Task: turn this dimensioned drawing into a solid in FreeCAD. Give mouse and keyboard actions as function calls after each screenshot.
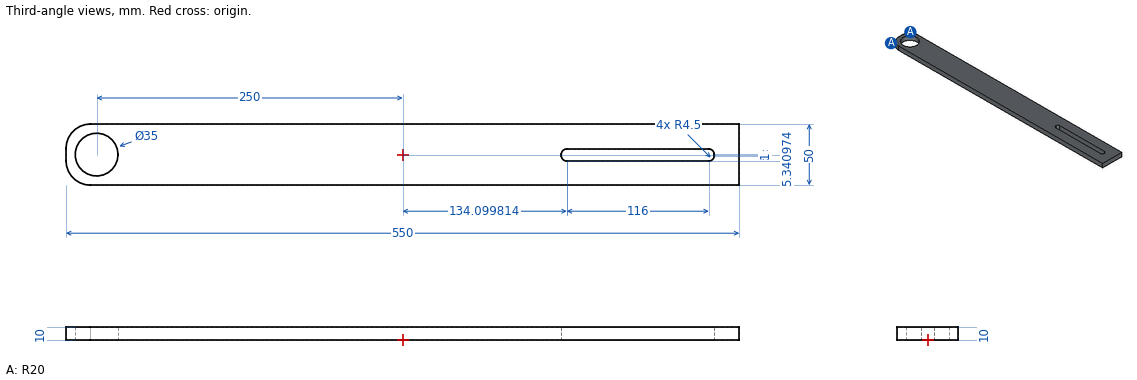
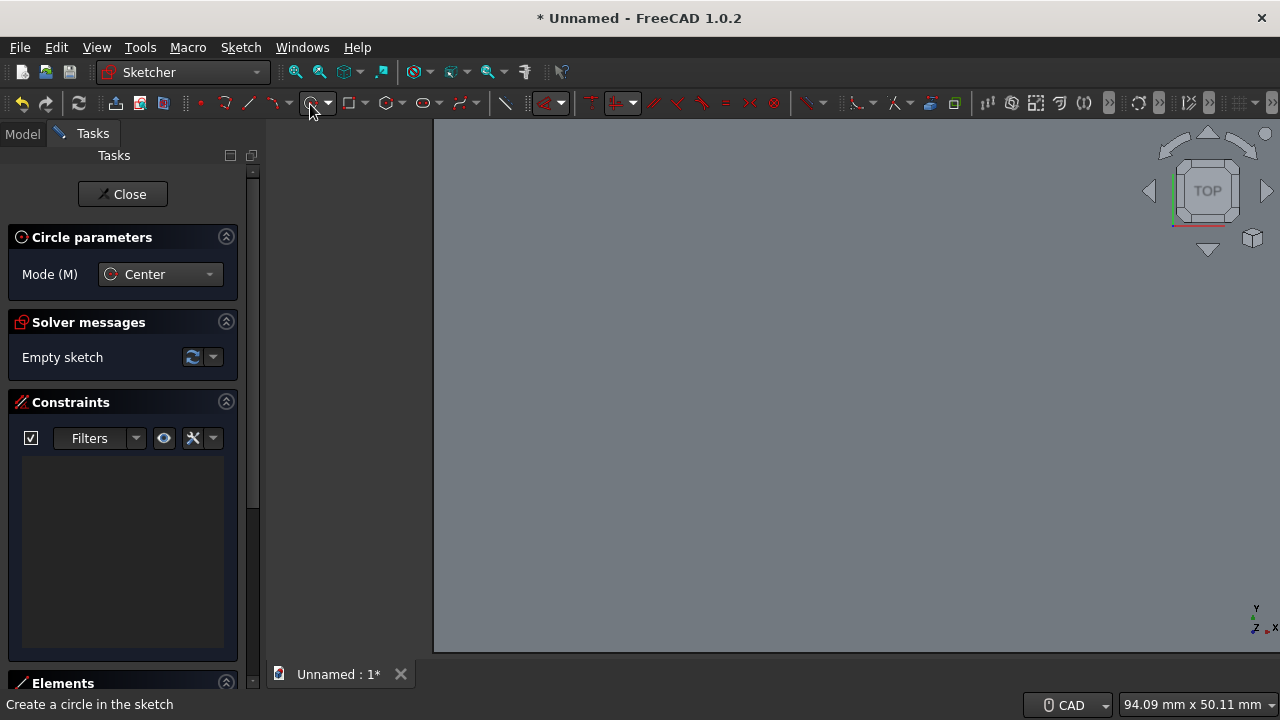
click(703, 384)
click(836, 251)
key(Escape)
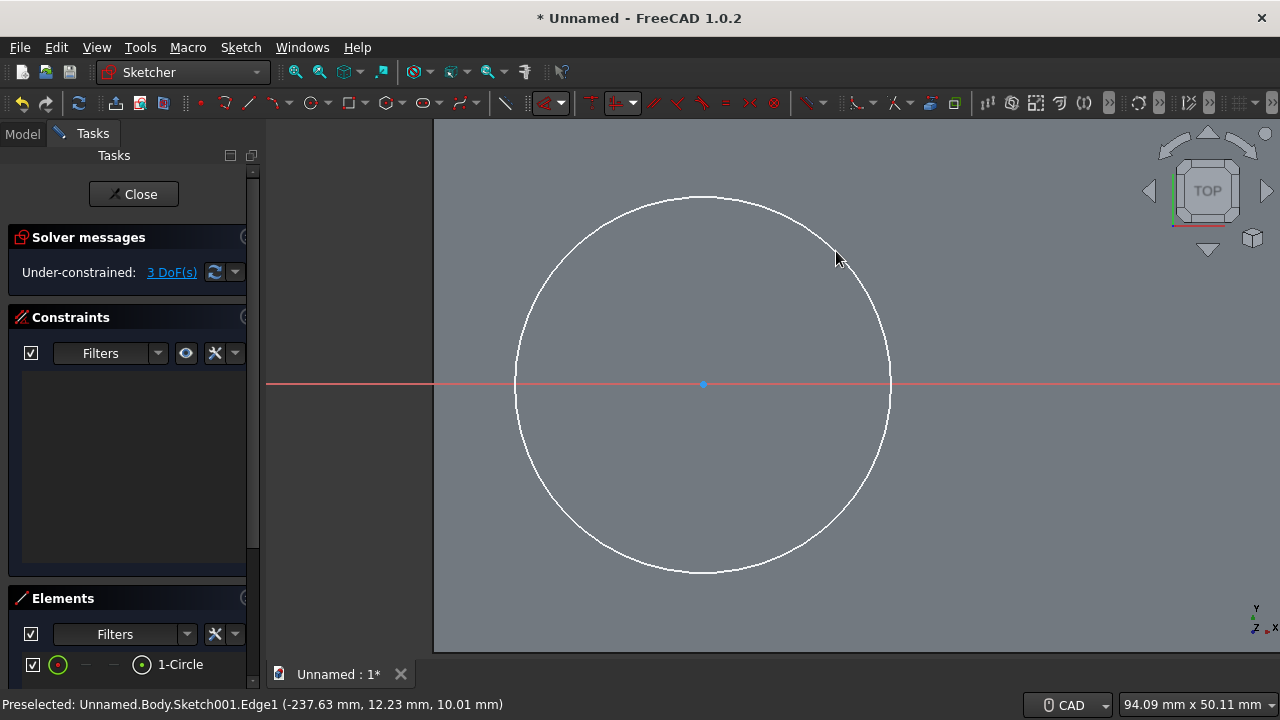
click(703, 385)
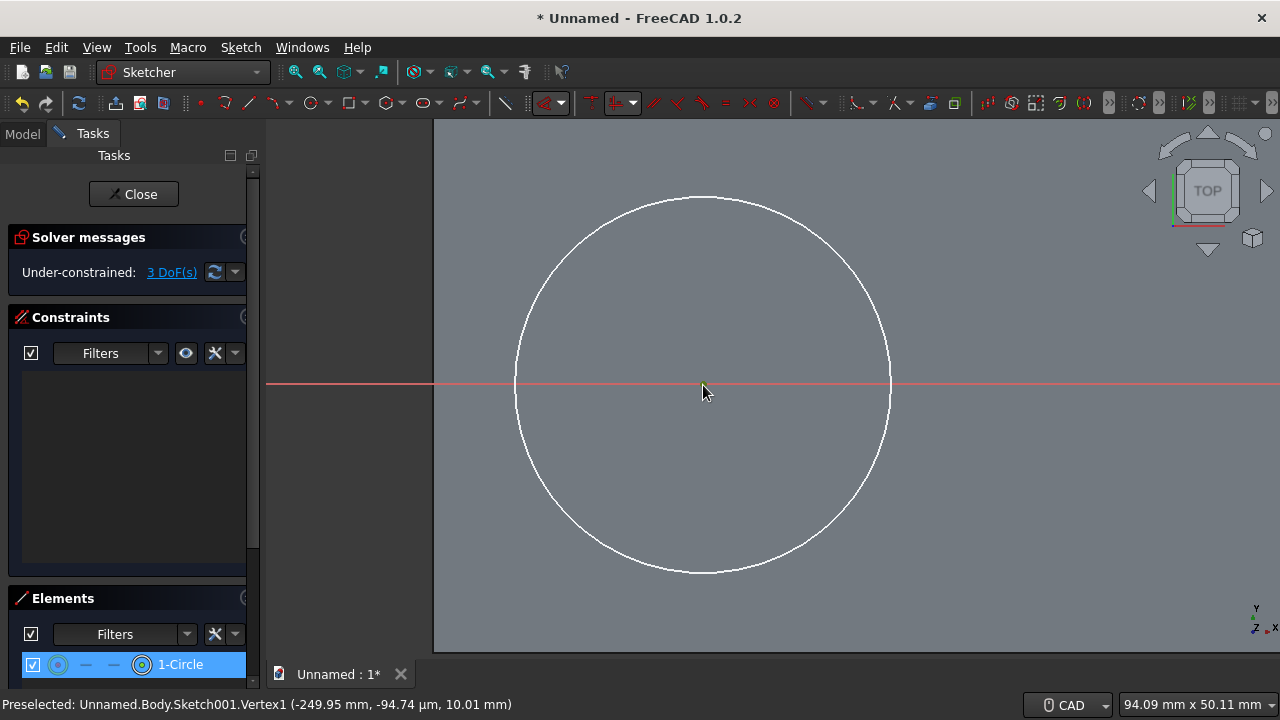
click(353, 384)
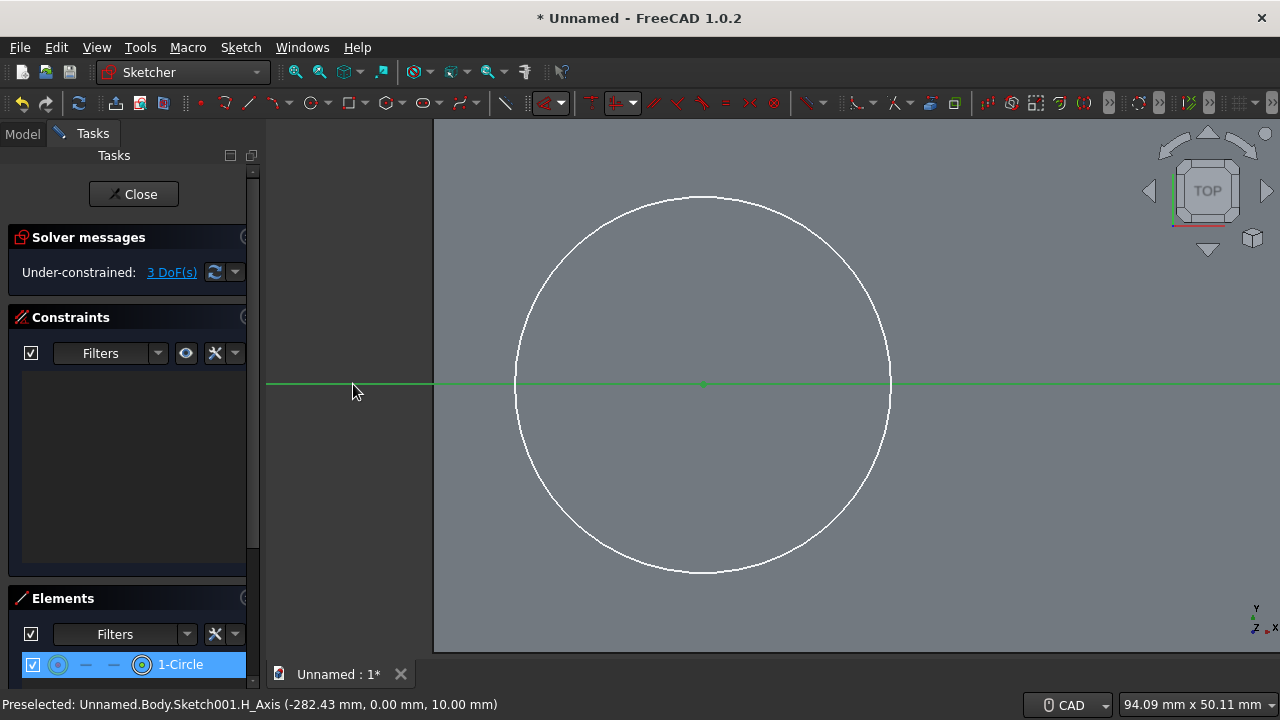
key(c)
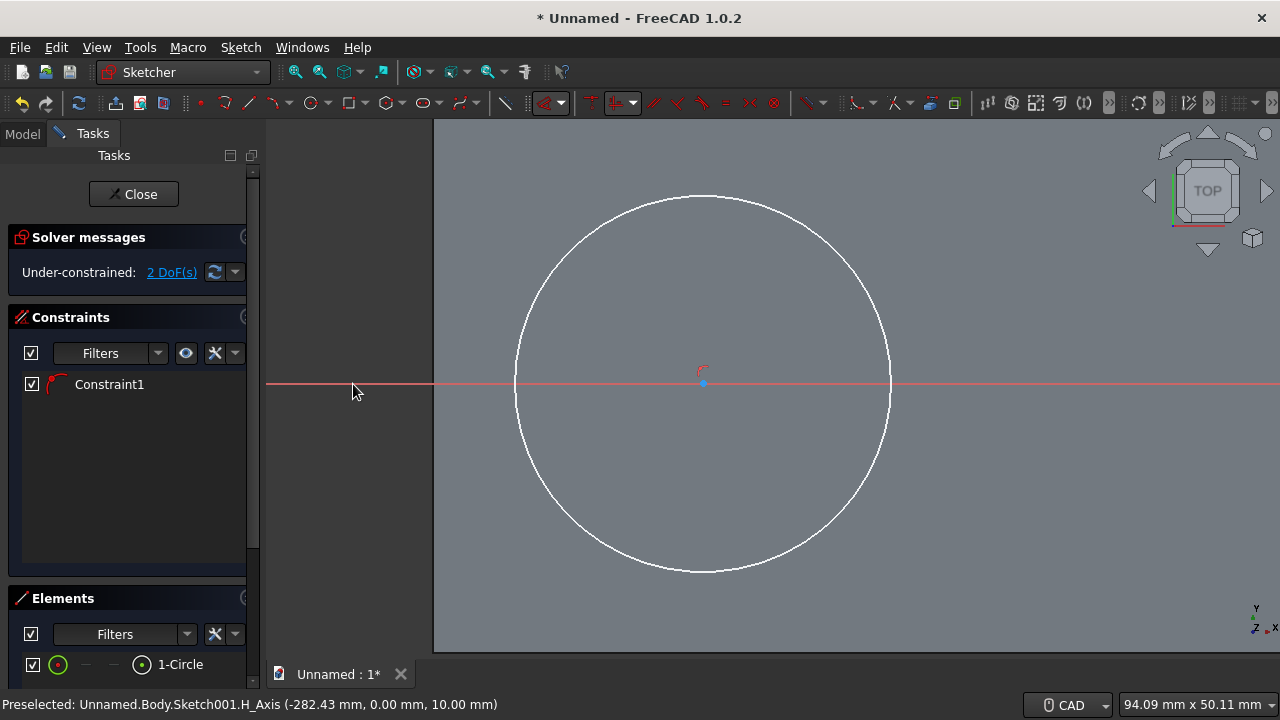
click(836, 251)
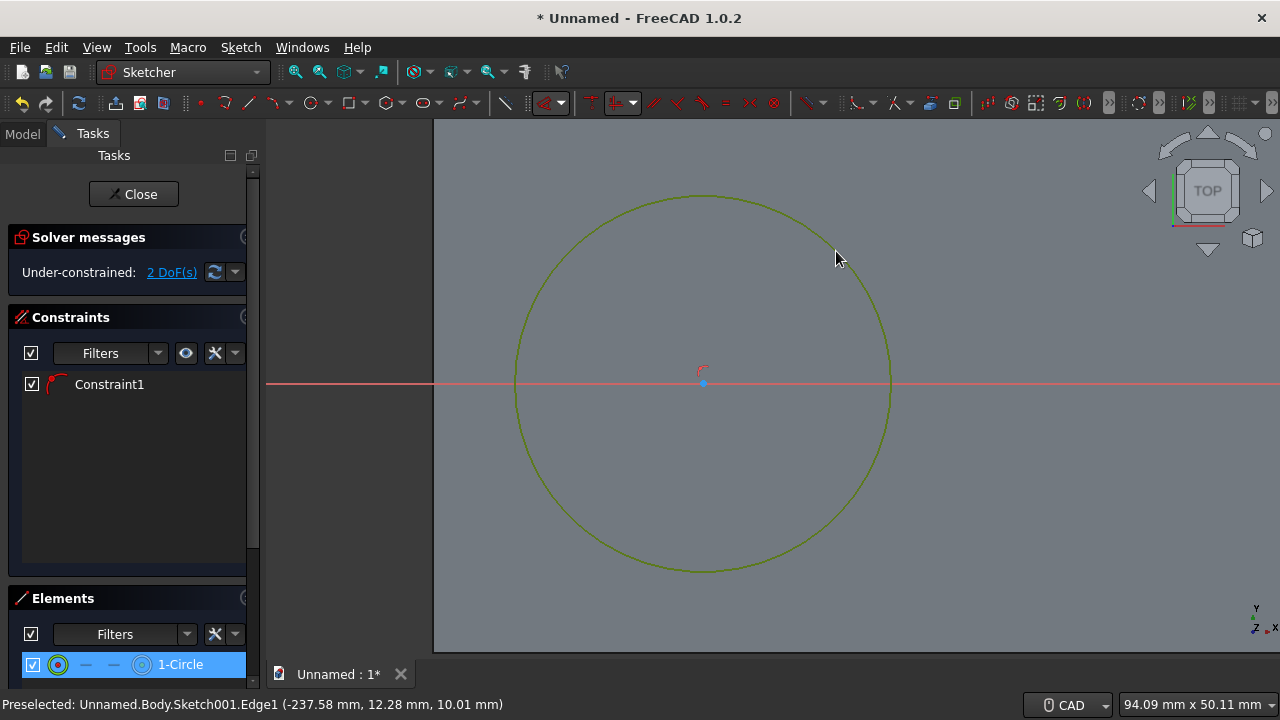
click(564, 104)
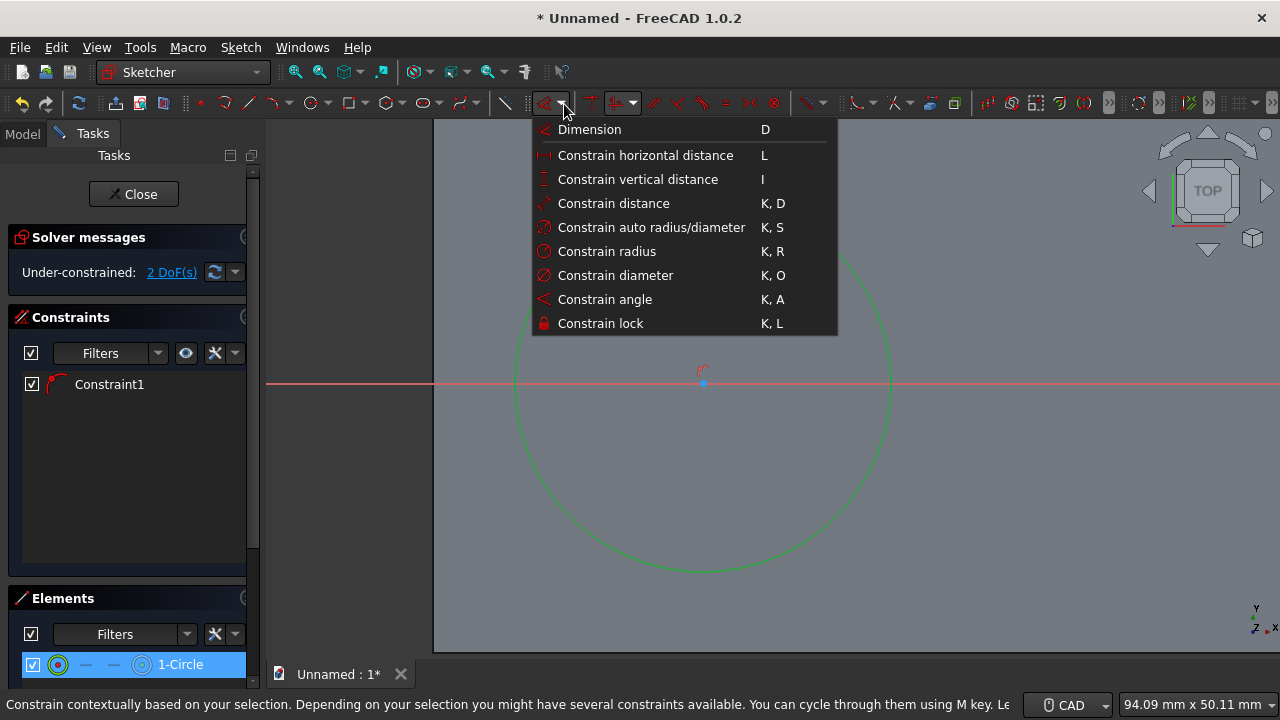
click(685, 275)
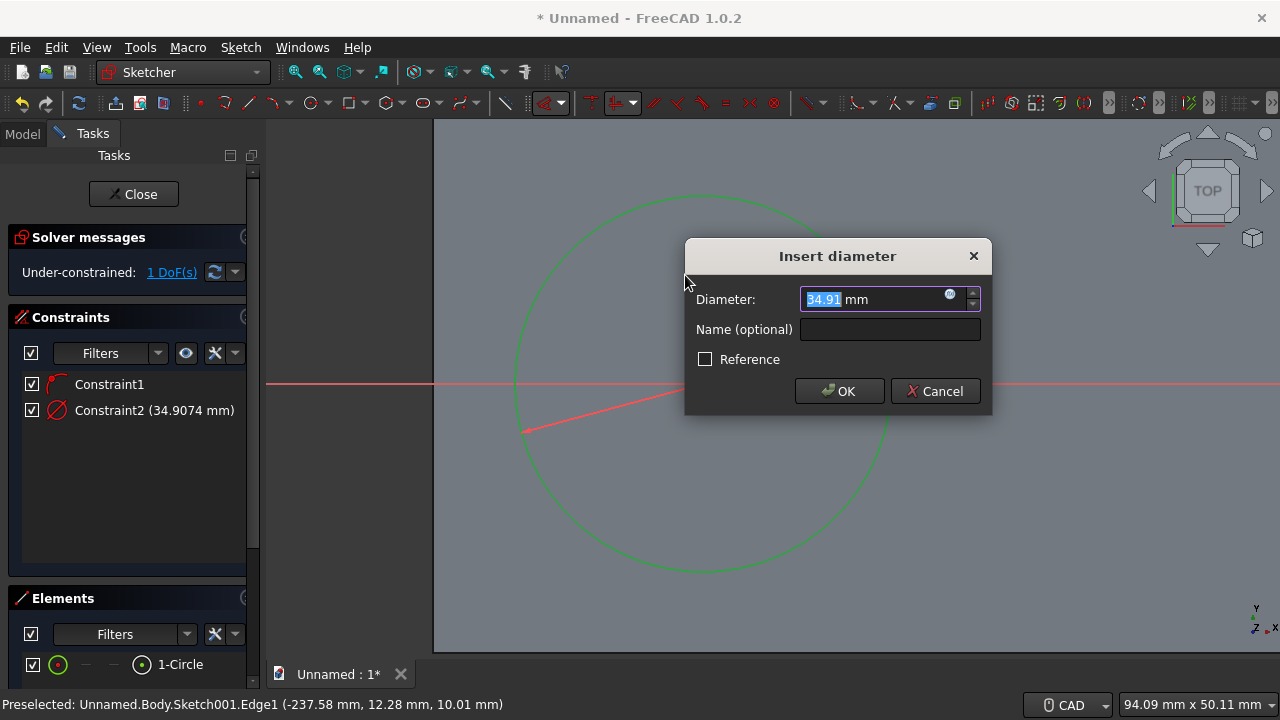
text(35)
key(Return)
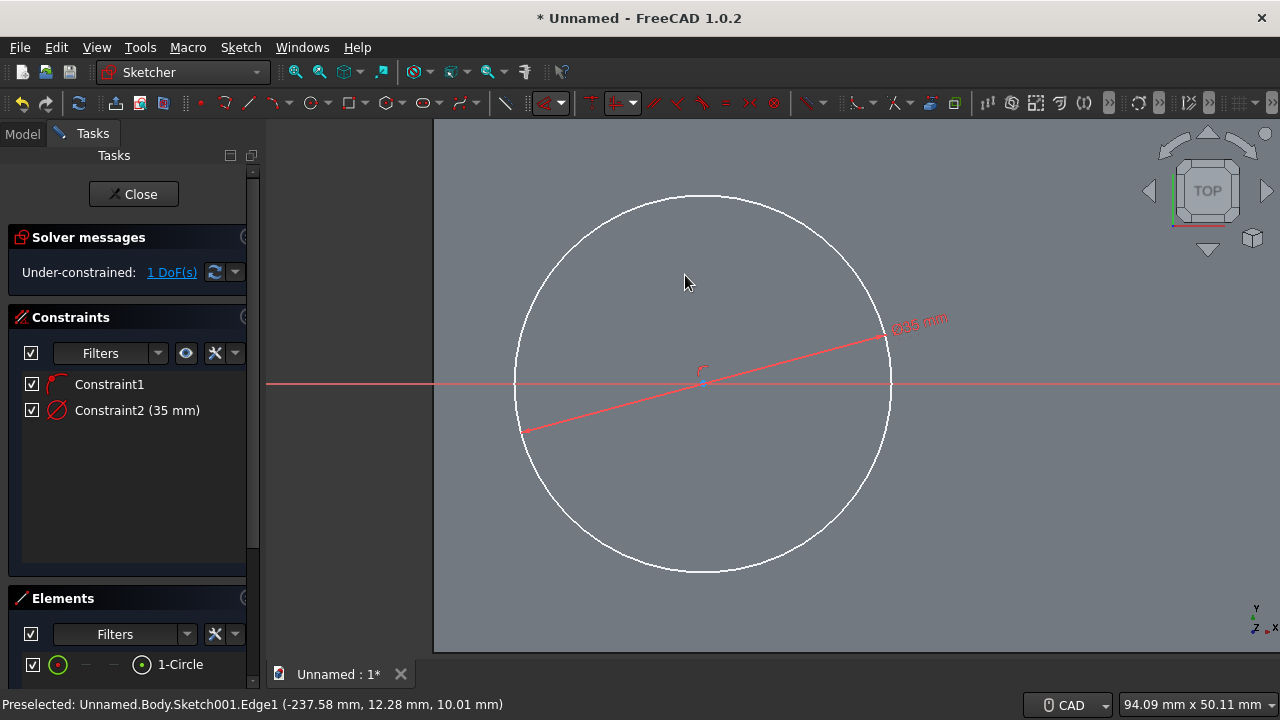
click(703, 384)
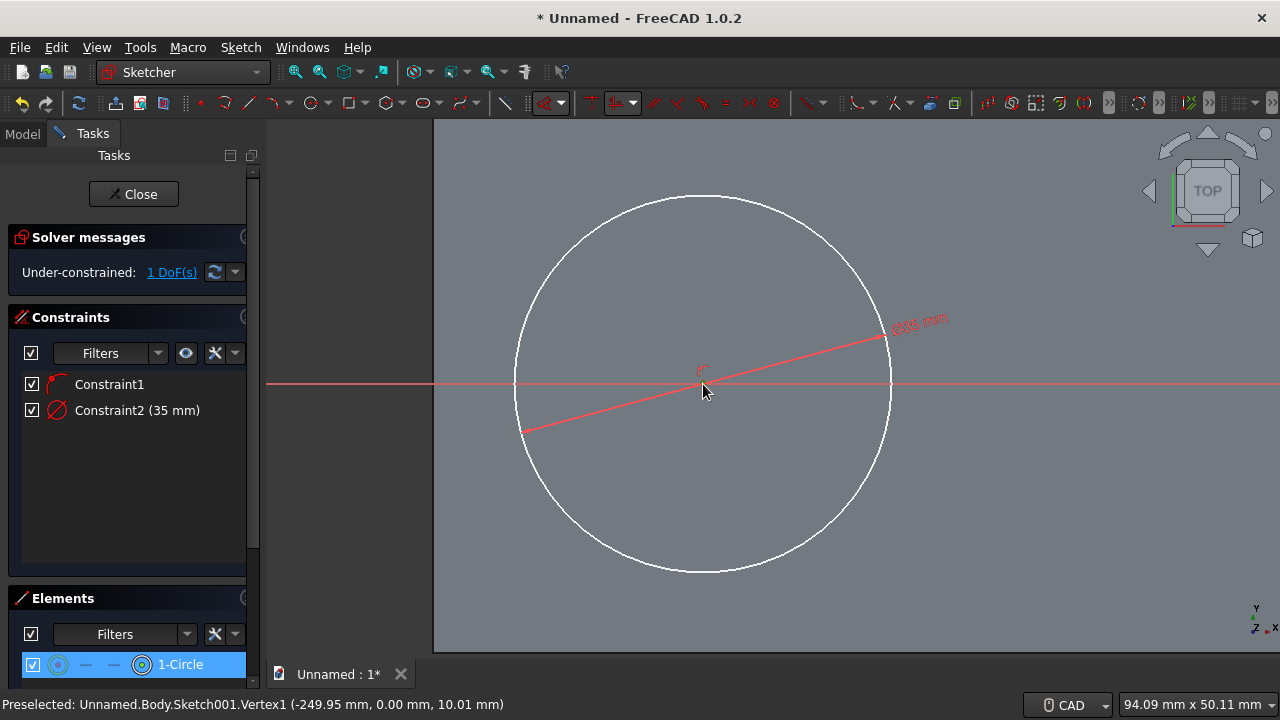
click(564, 104)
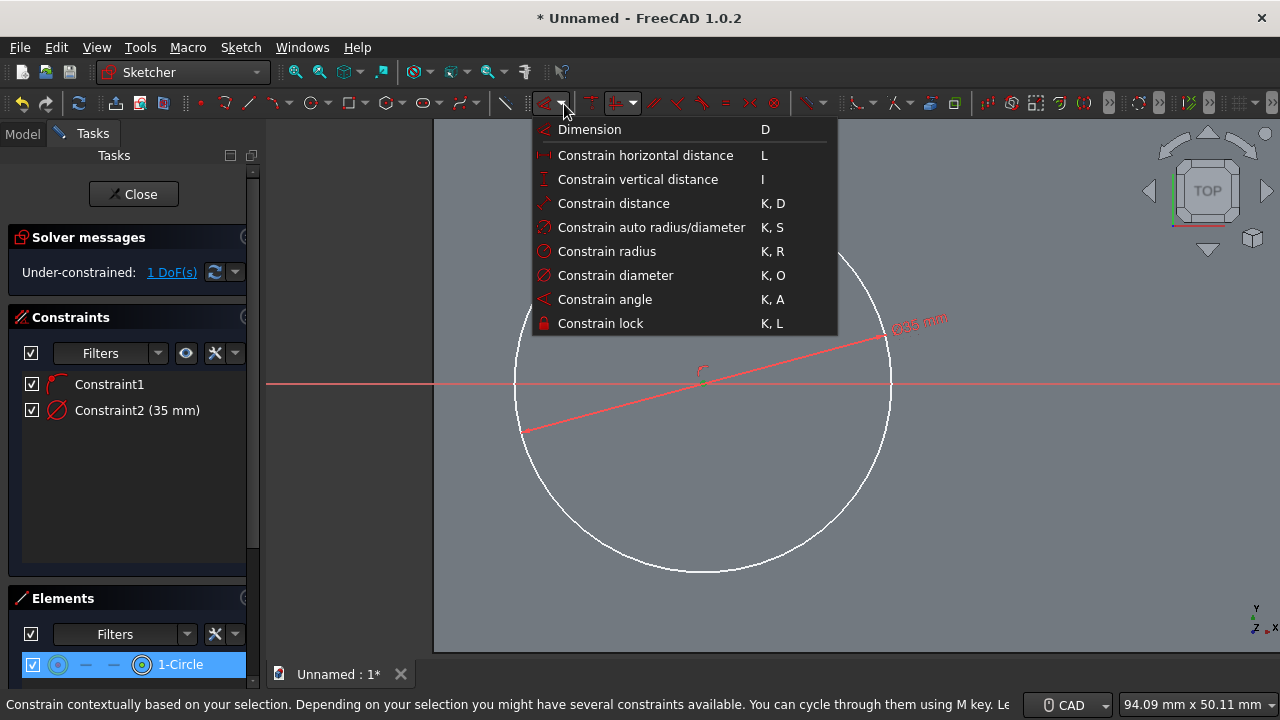
click(685, 155)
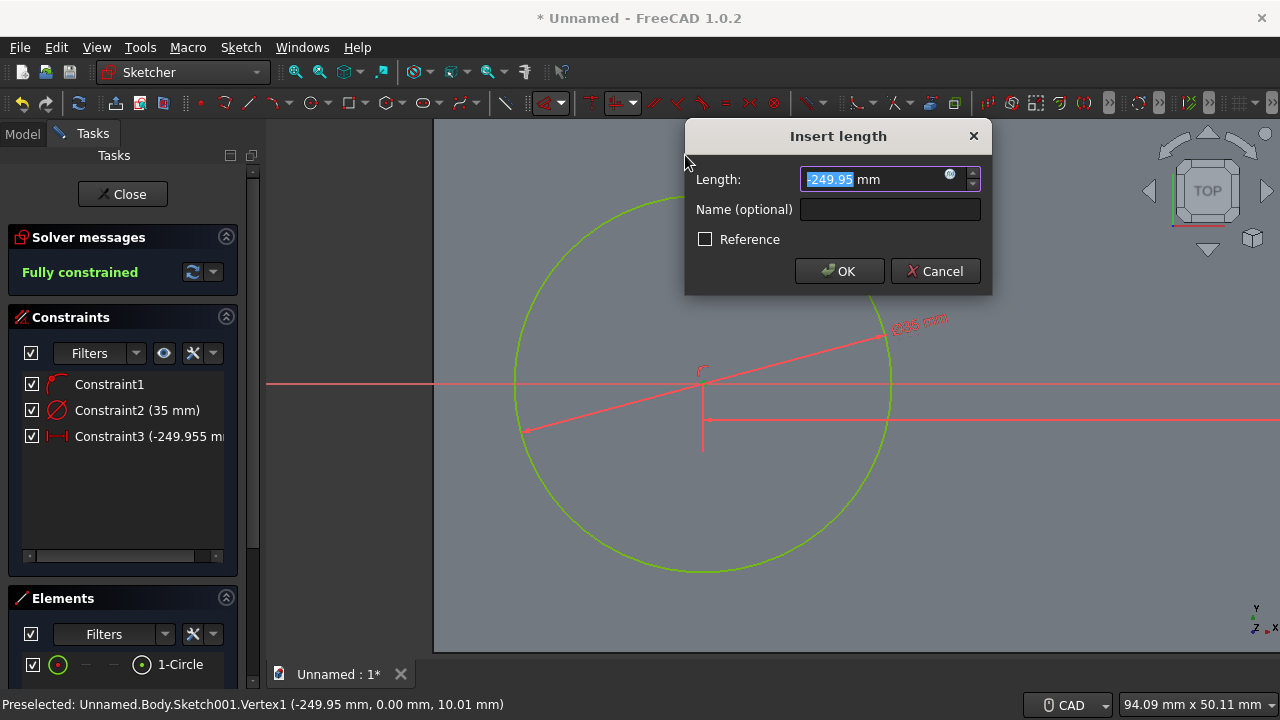
text(-250)
key(Return)